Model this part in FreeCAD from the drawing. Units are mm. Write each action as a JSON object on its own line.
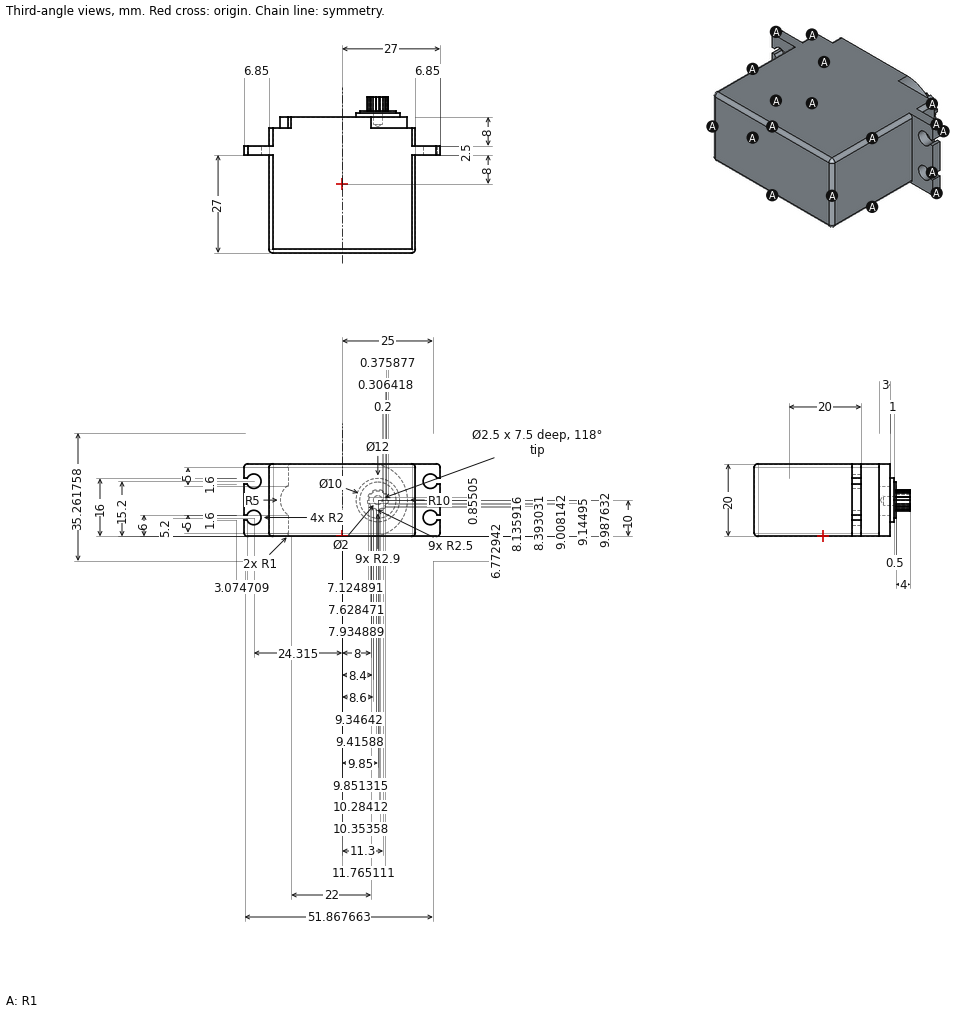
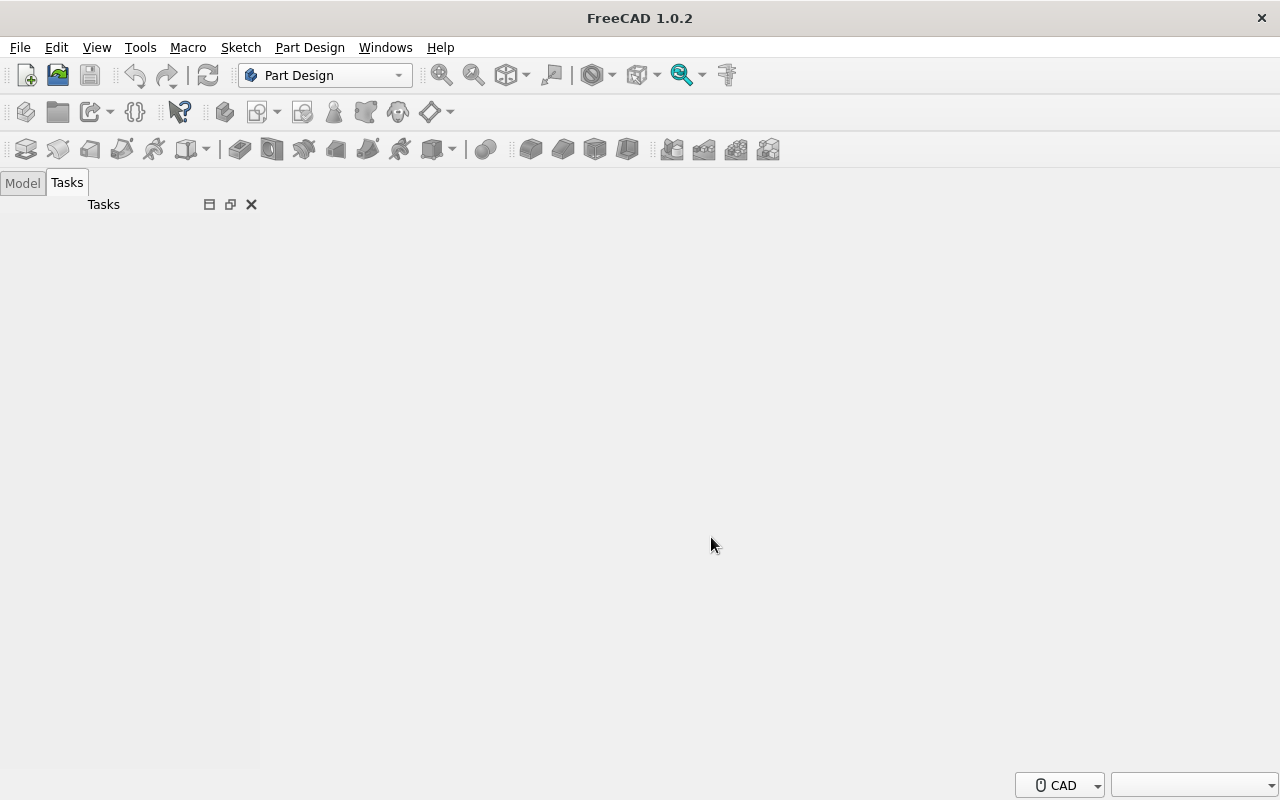
{"action": "left_click", "coordinate": [26, 76]}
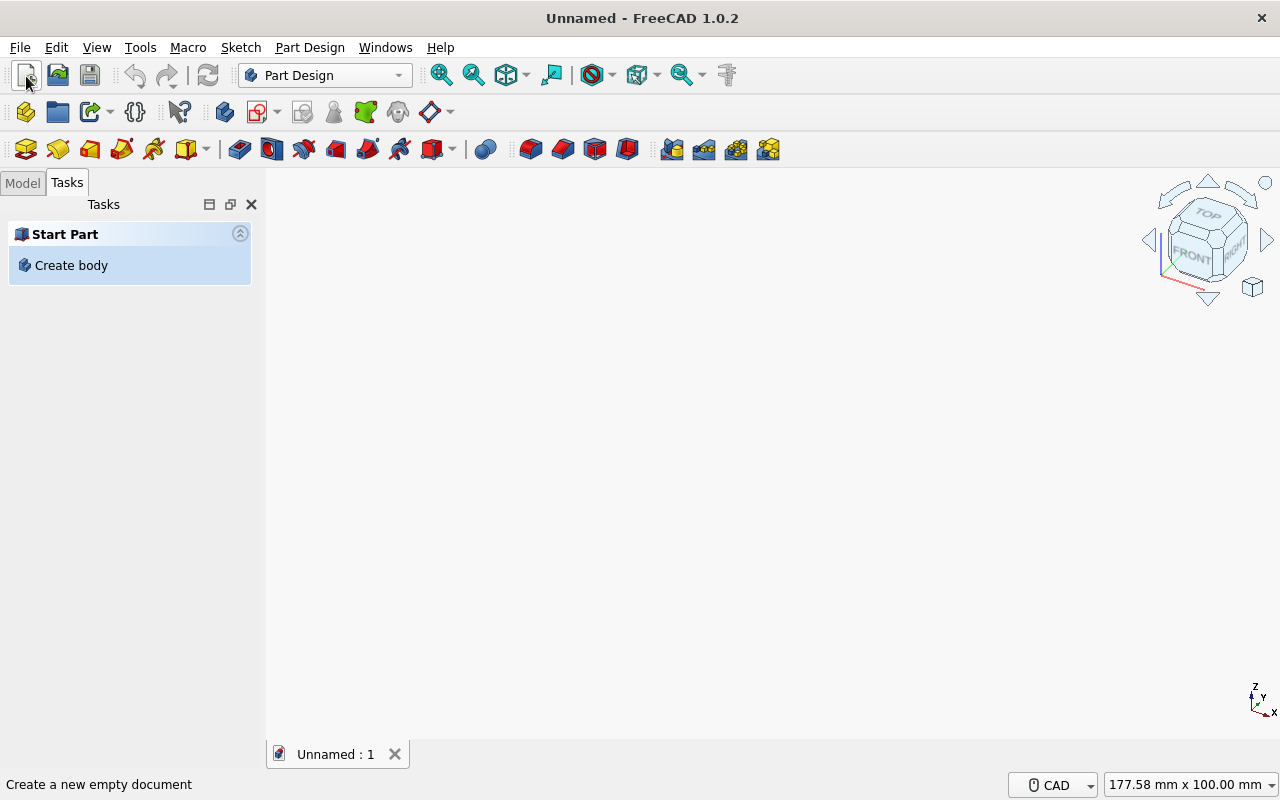
{"action": "left_click", "coordinate": [258, 112]}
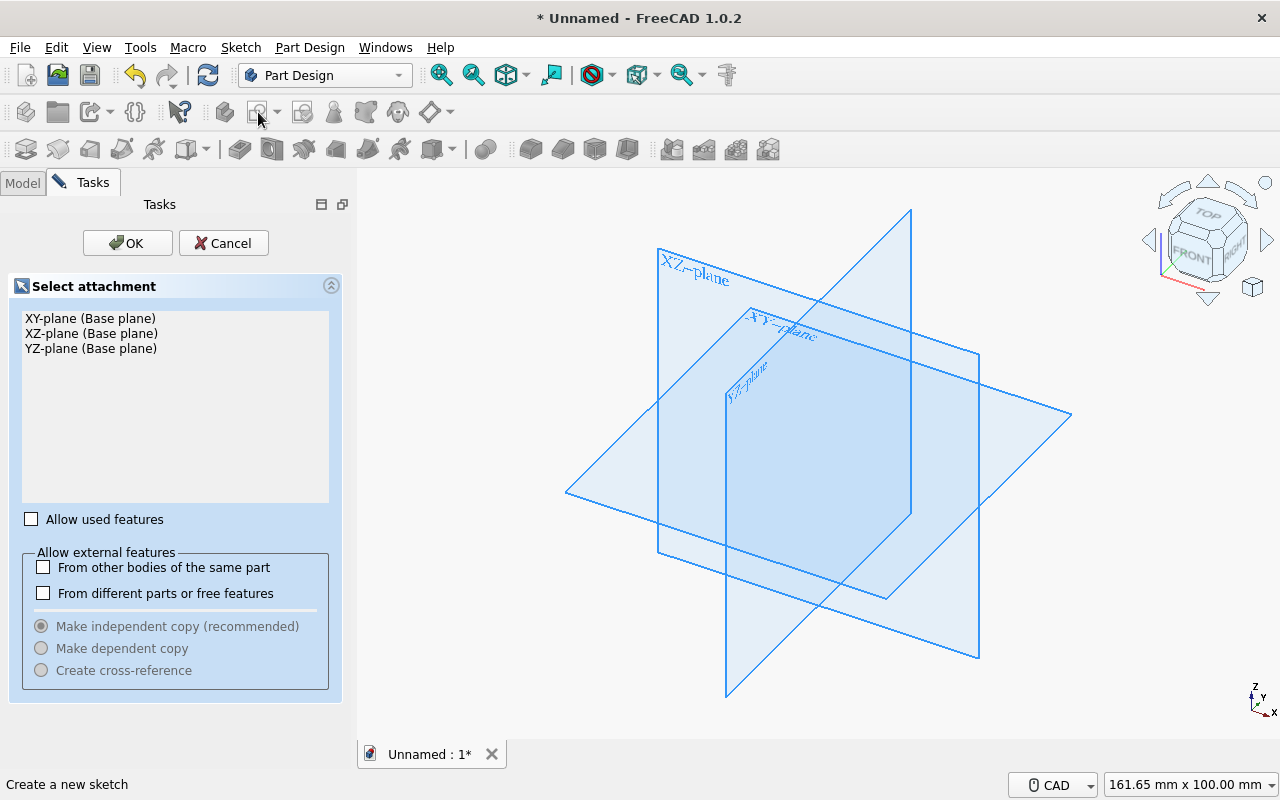
{"action": "left_click", "coordinate": [82, 318]}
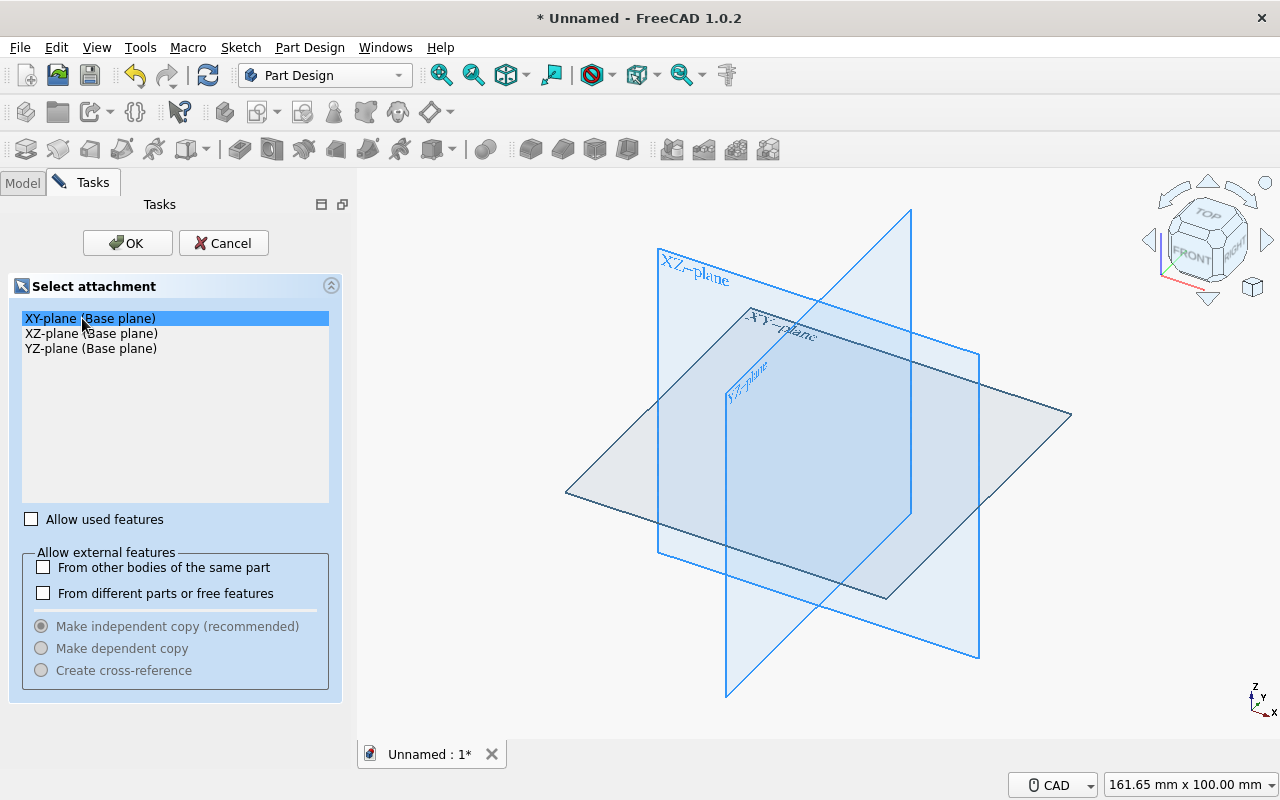
{"action": "left_click", "coordinate": [128, 243]}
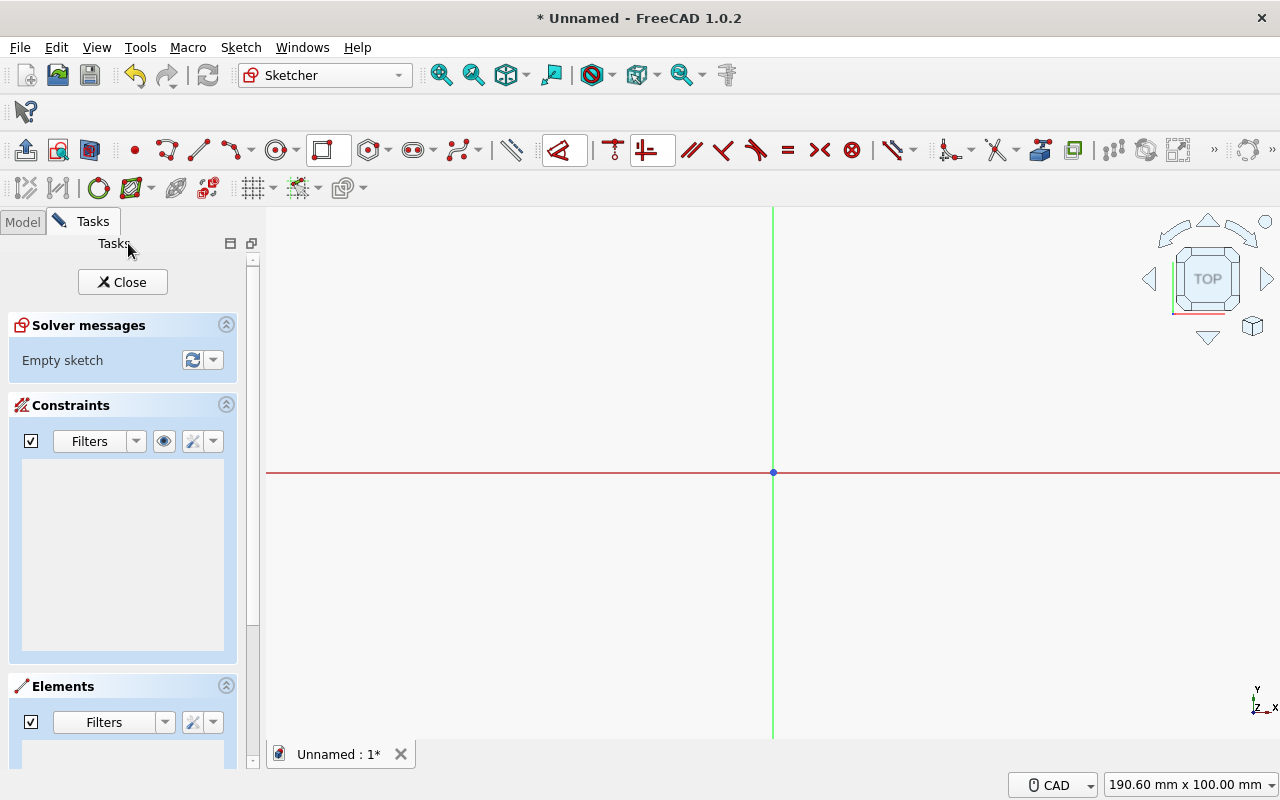
{"action": "scroll", "coordinate": [856, 476], "scroll_direction": "up", "scroll_amount": 3}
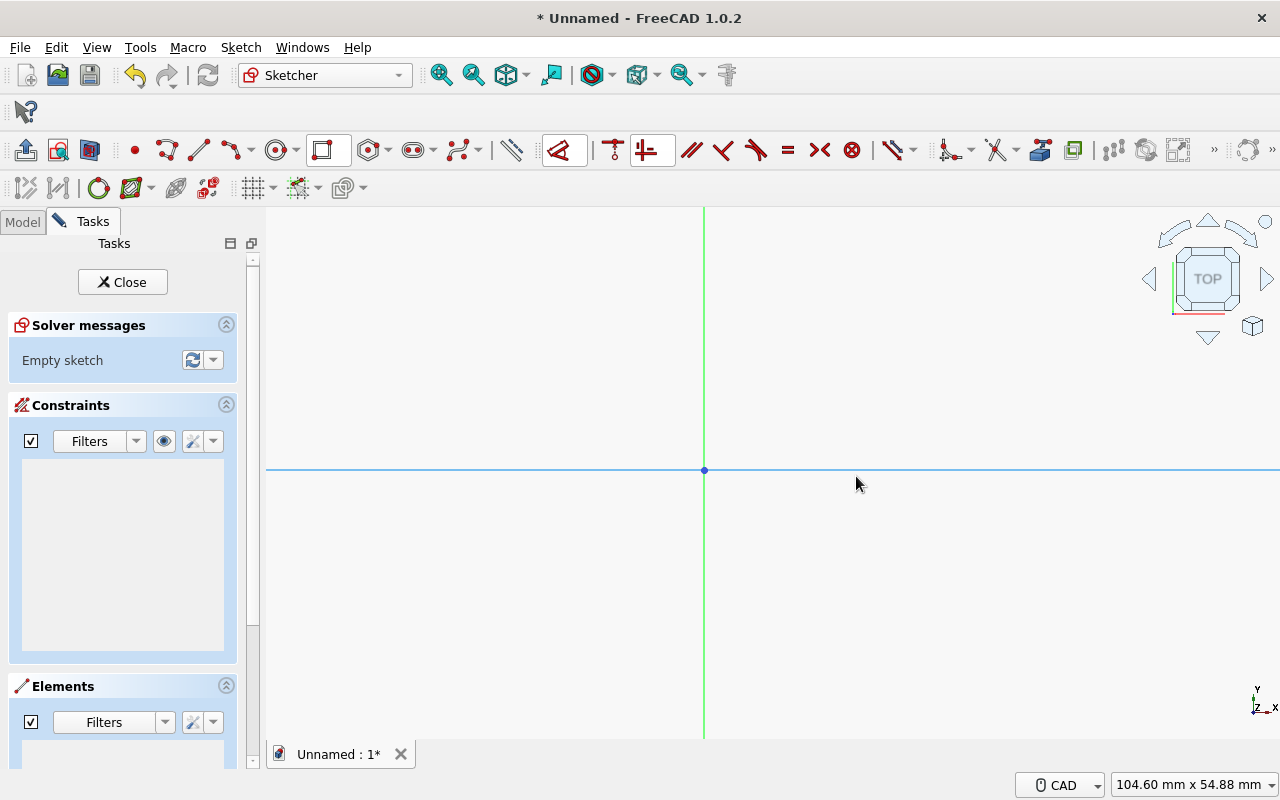
{"action": "left_click", "coordinate": [168, 150]}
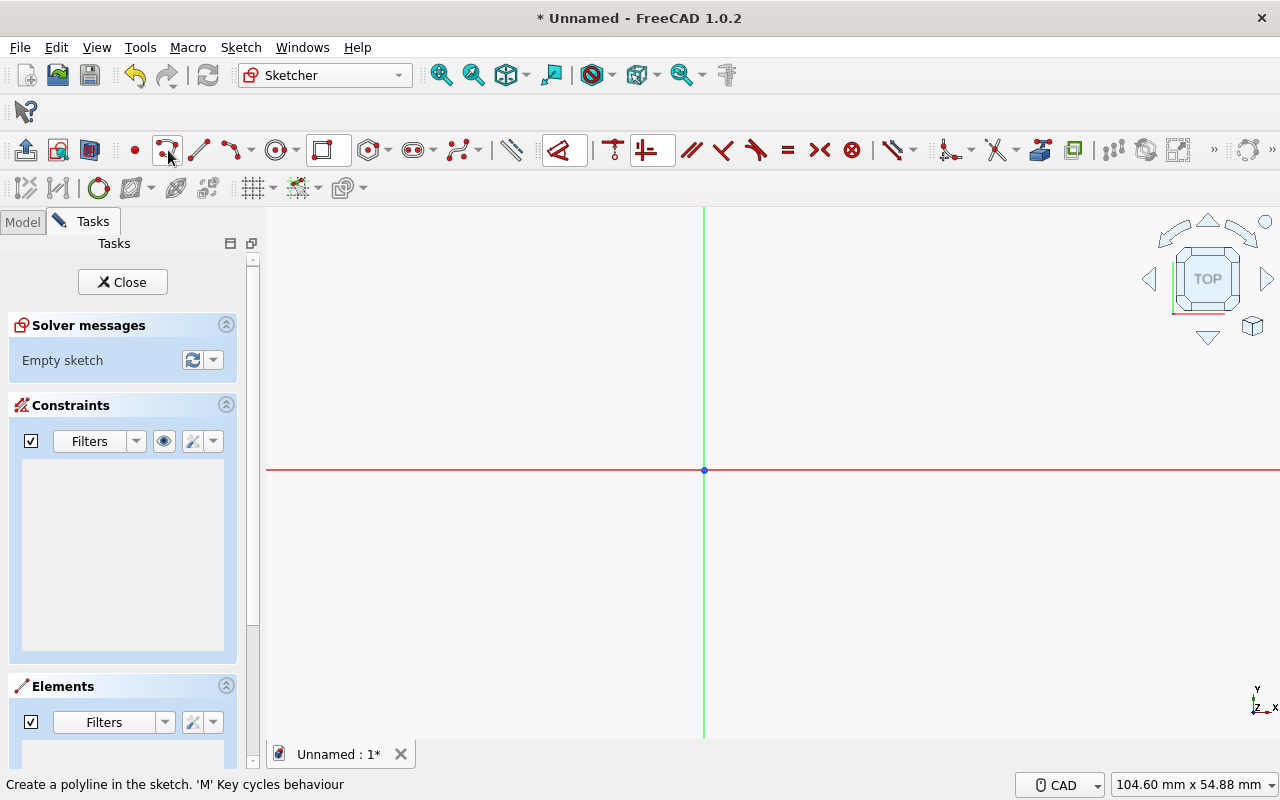
{"action": "left_click", "coordinate": [900, 393]}
{"action": "left_click", "coordinate": [966, 393]}
{"action": "left_click", "coordinate": [966, 368]}
{"action": "left_click", "coordinate": [900, 368]}
{"action": "left_click", "coordinate": [900, 291]}
{"action": "left_click", "coordinate": [509, 291]}
{"action": "left_click", "coordinate": [509, 368]}
{"action": "left_click", "coordinate": [443, 368]}
{"action": "left_click", "coordinate": [443, 393]}
{"action": "left_click", "coordinate": [509, 393]}
{"action": "left_click", "coordinate": [509, 654]}
{"action": "left_click", "coordinate": [900, 654]}
{"action": "left_click", "coordinate": [900, 394]}
{"action": "key", "text": "Escape"}
{"action": "key", "text": "Escape"}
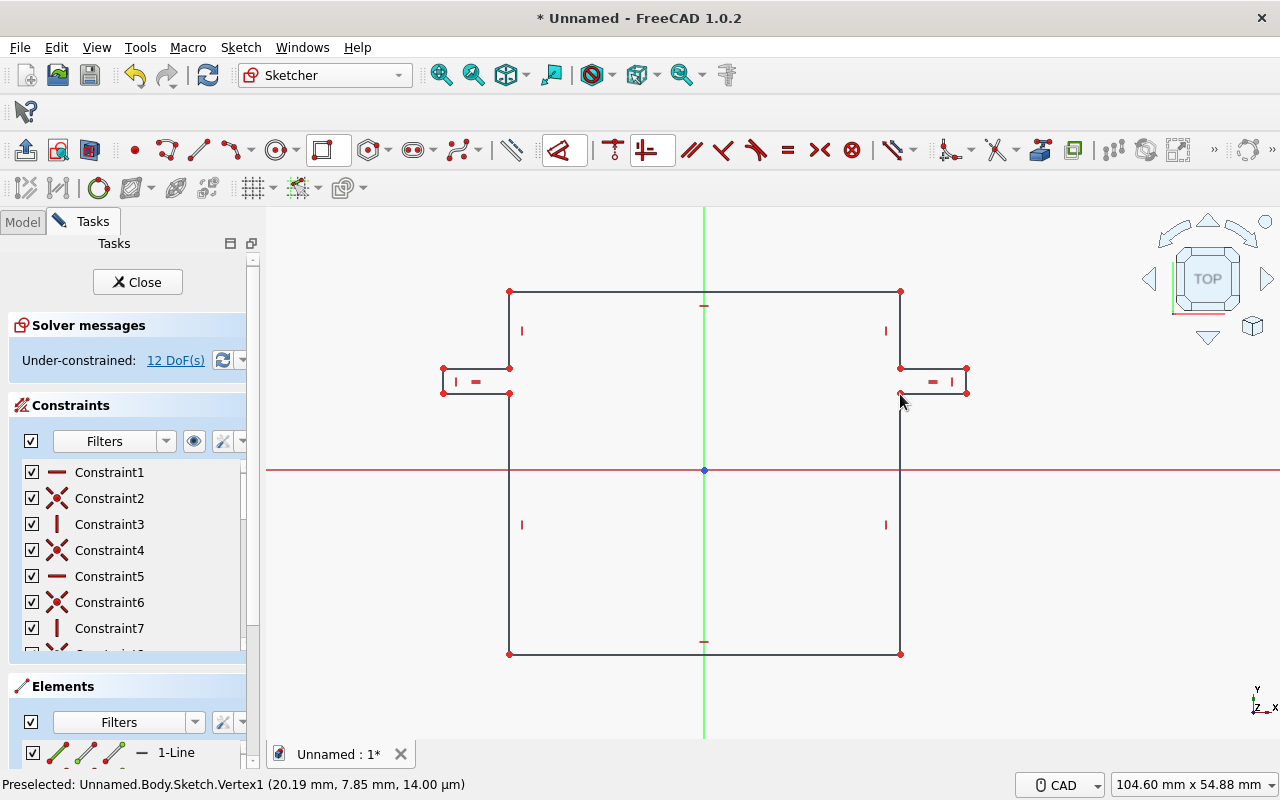
{"action": "left_click", "coordinate": [900, 369]}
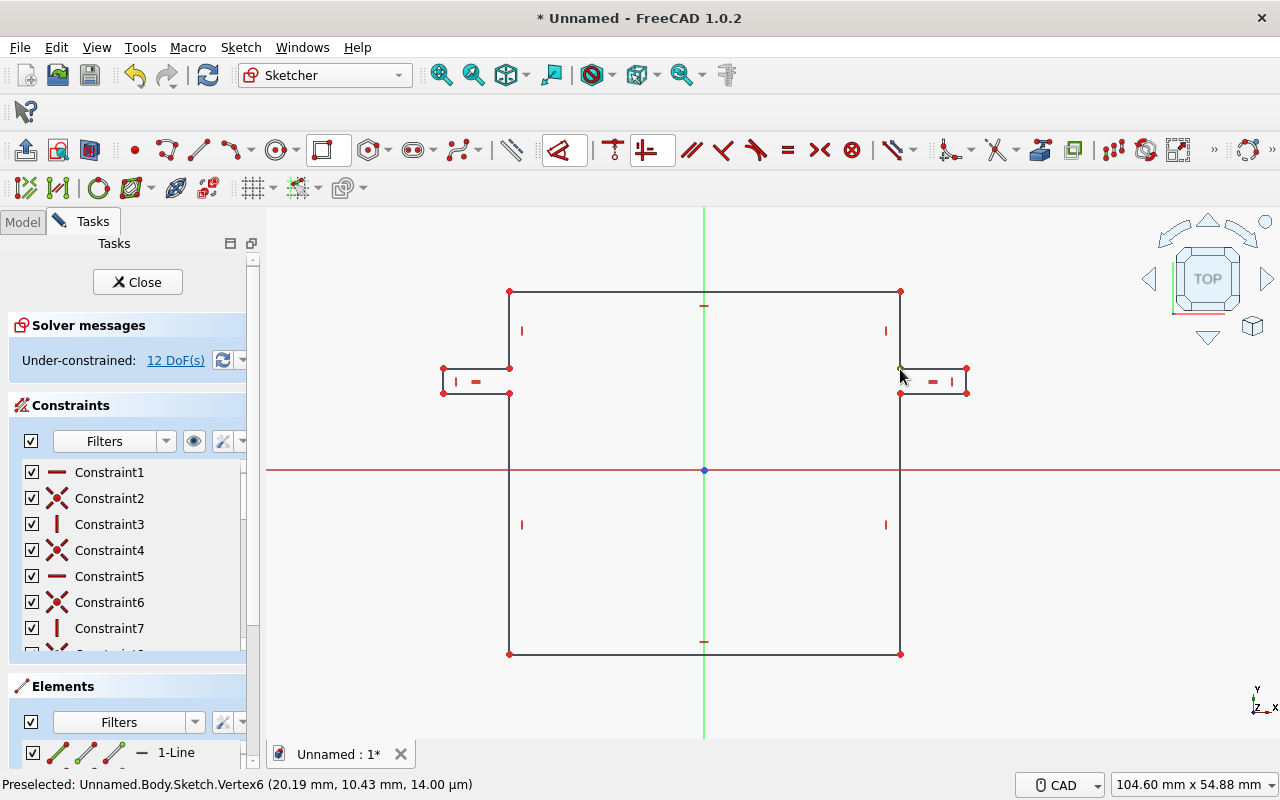
{"action": "left_click", "coordinate": [509, 369]}